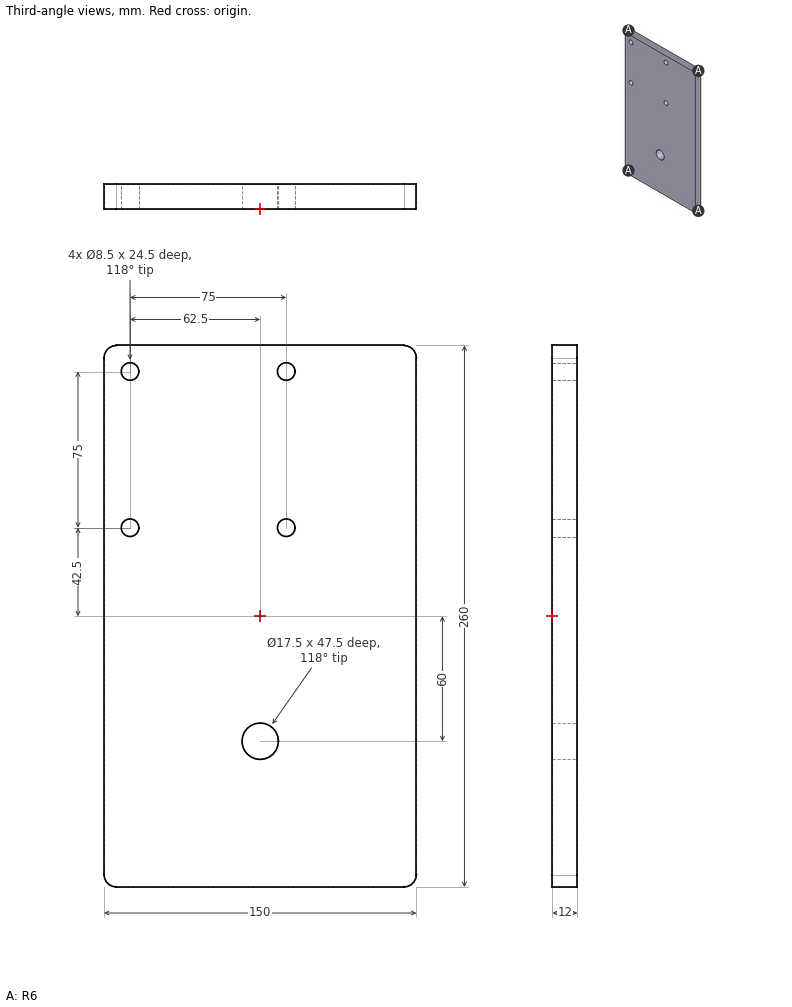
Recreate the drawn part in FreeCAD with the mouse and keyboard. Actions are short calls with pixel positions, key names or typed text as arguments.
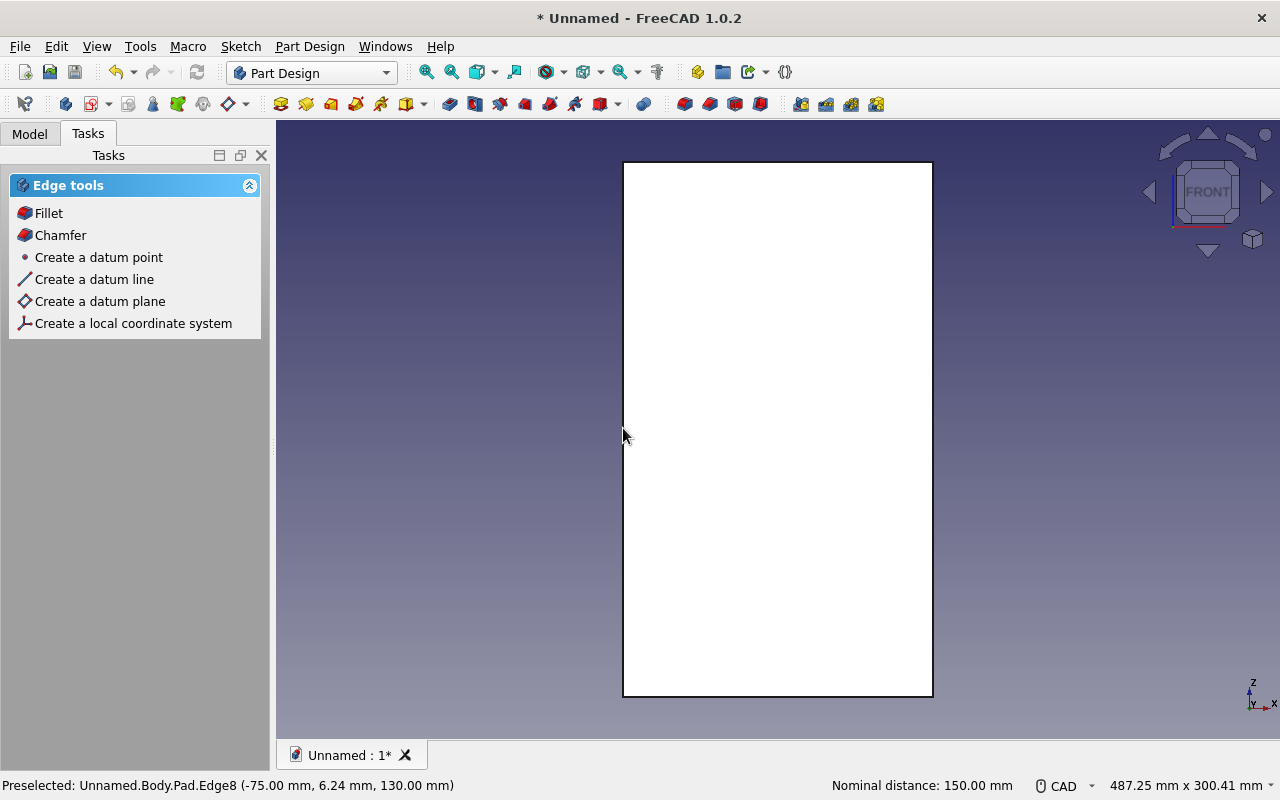
key(3)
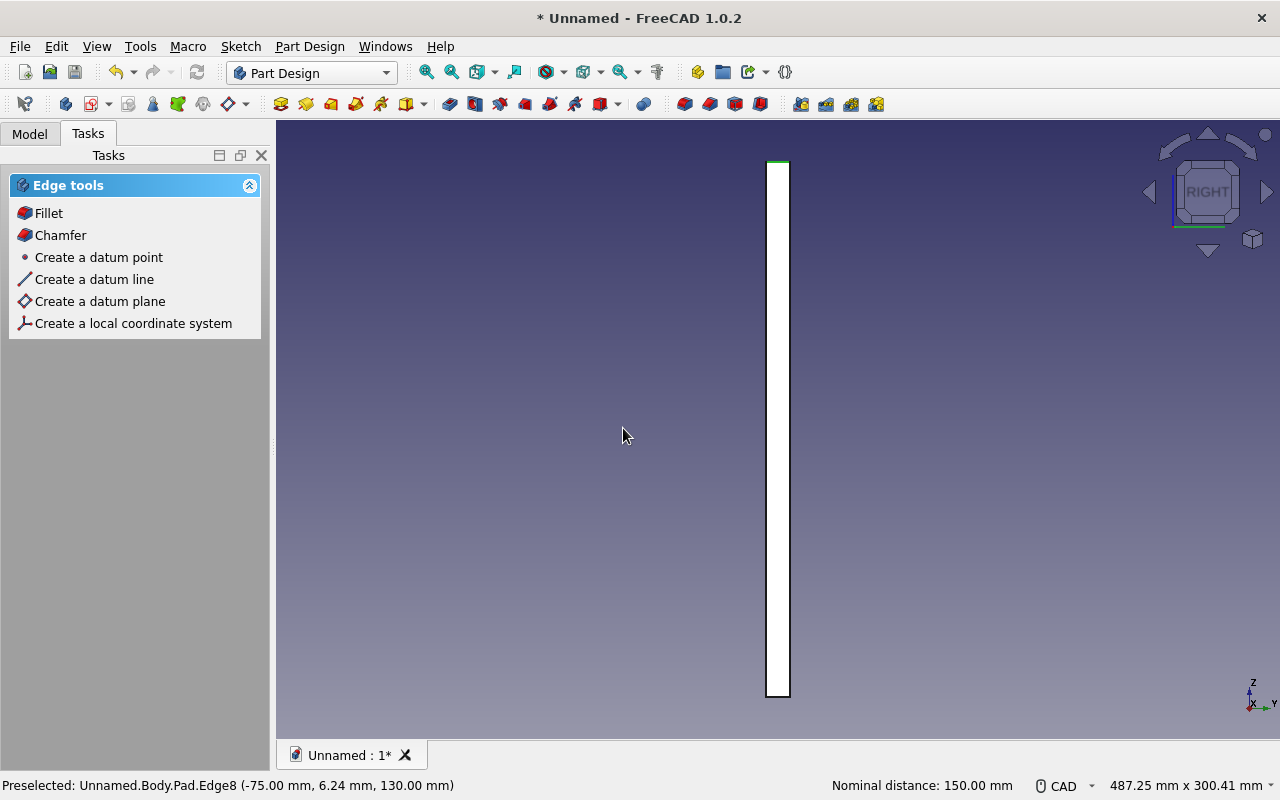
click(778, 696, ctrl)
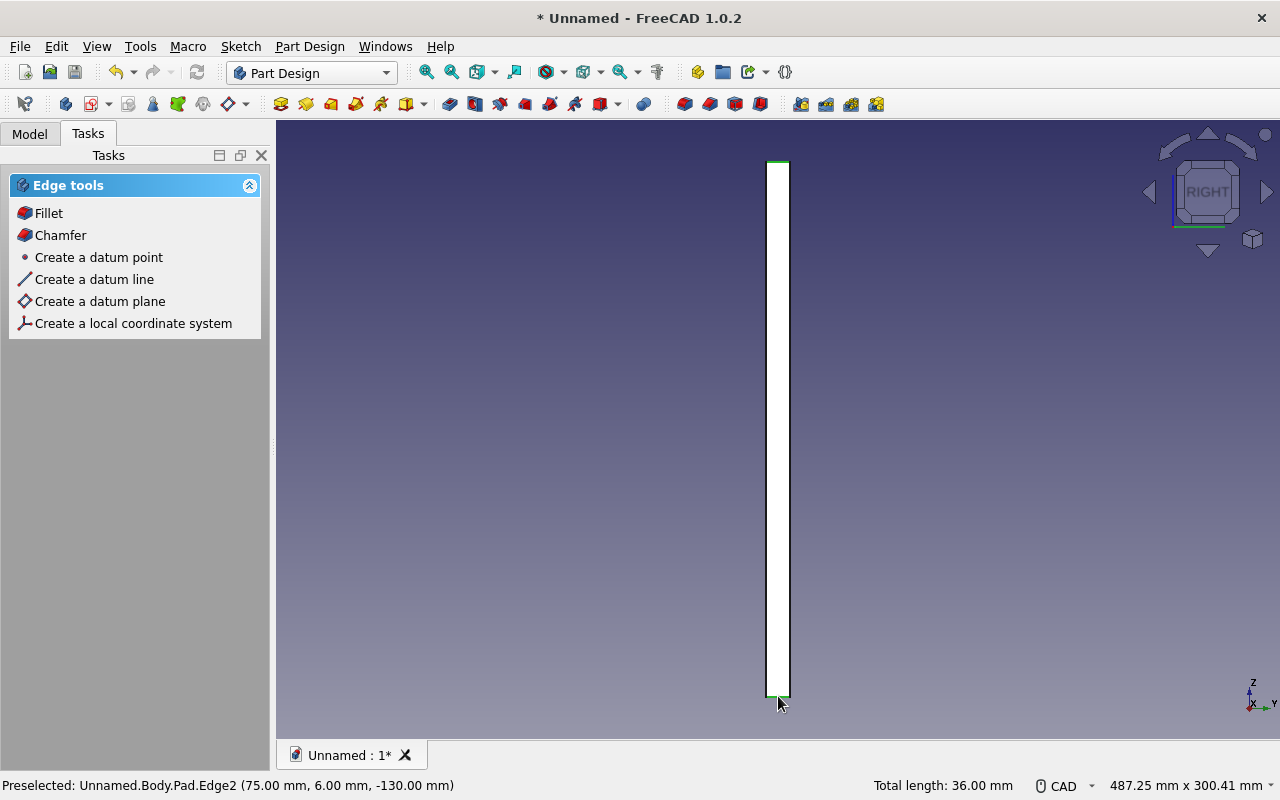
key(5)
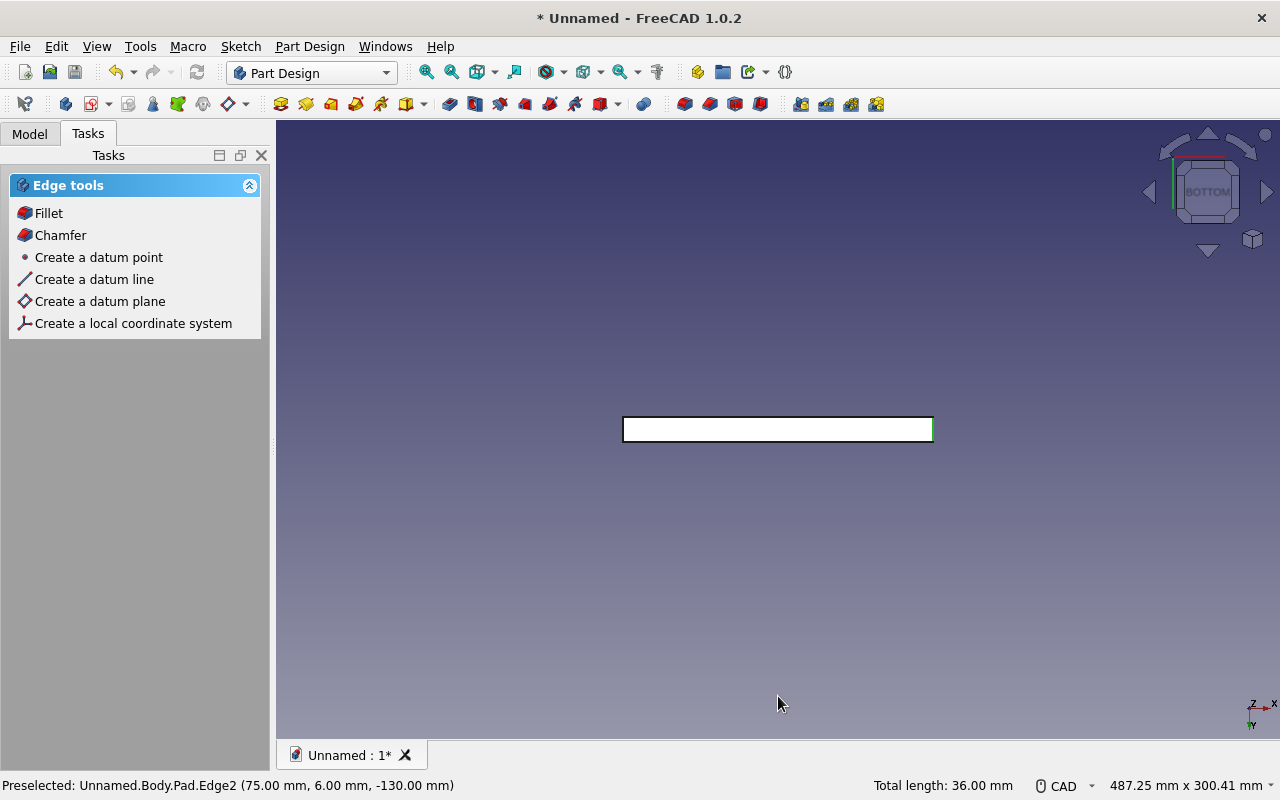
key(v)
key(f)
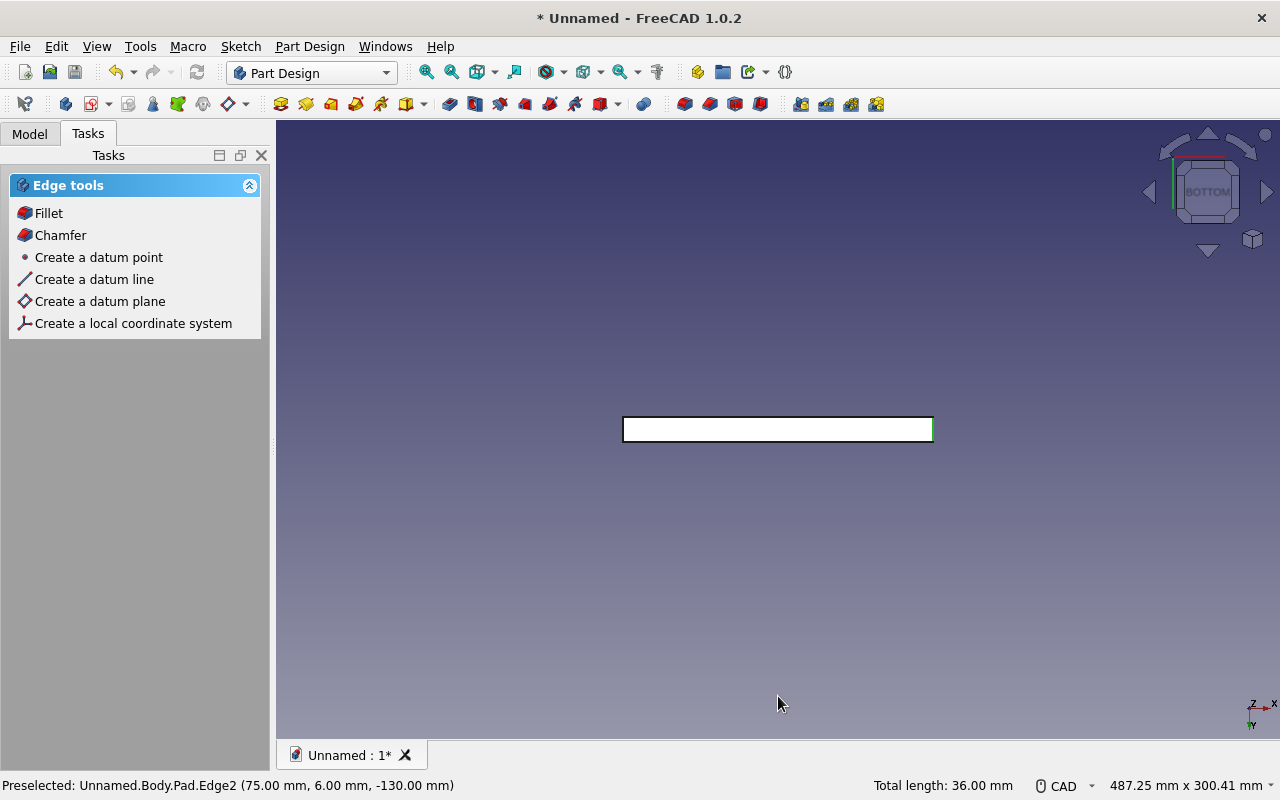
click(623, 428, ctrl)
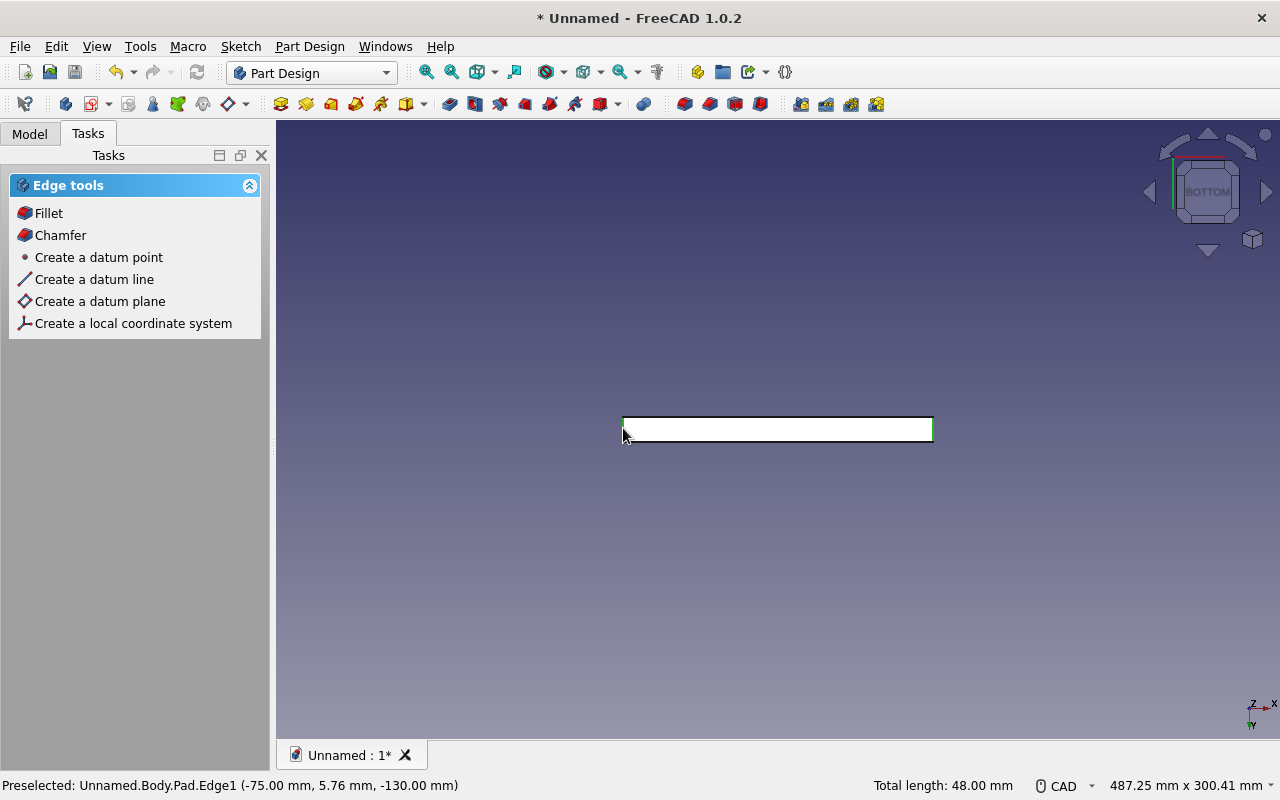
click(685, 104)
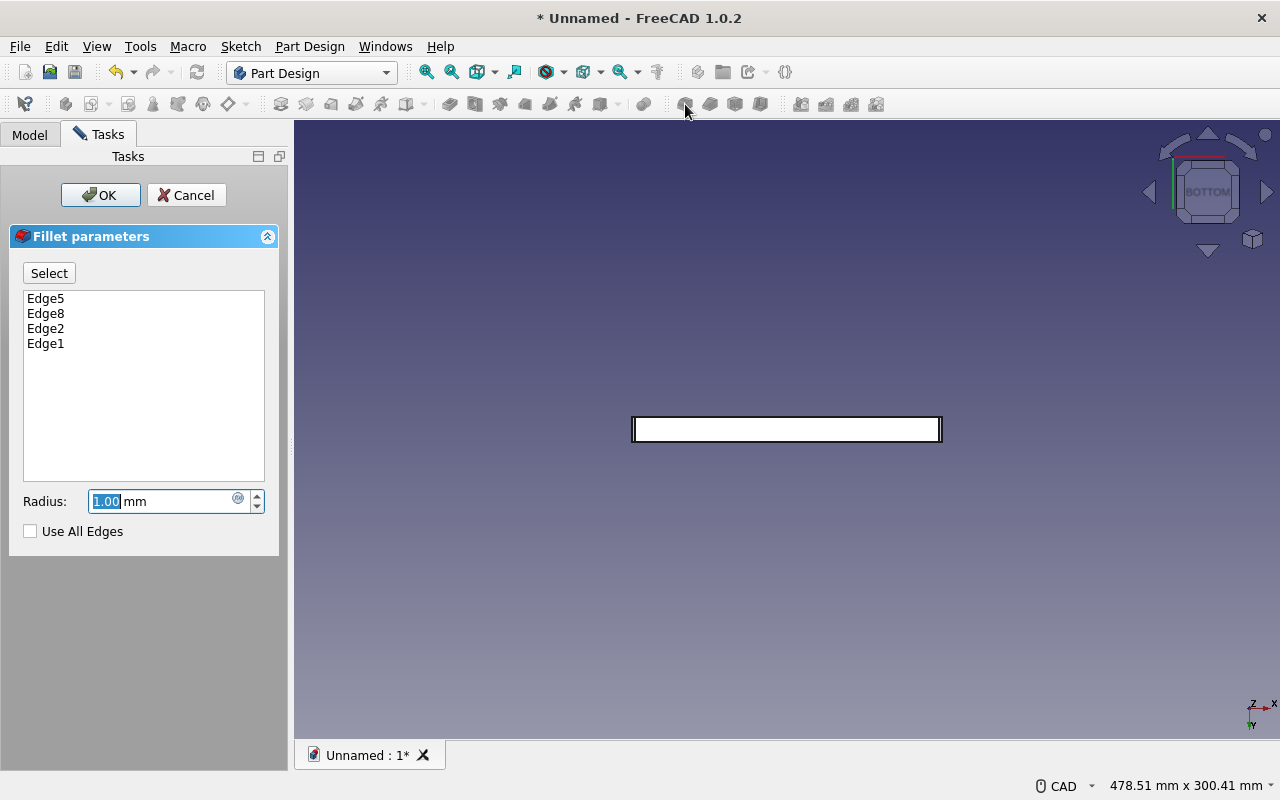
text(6)
key(Tab)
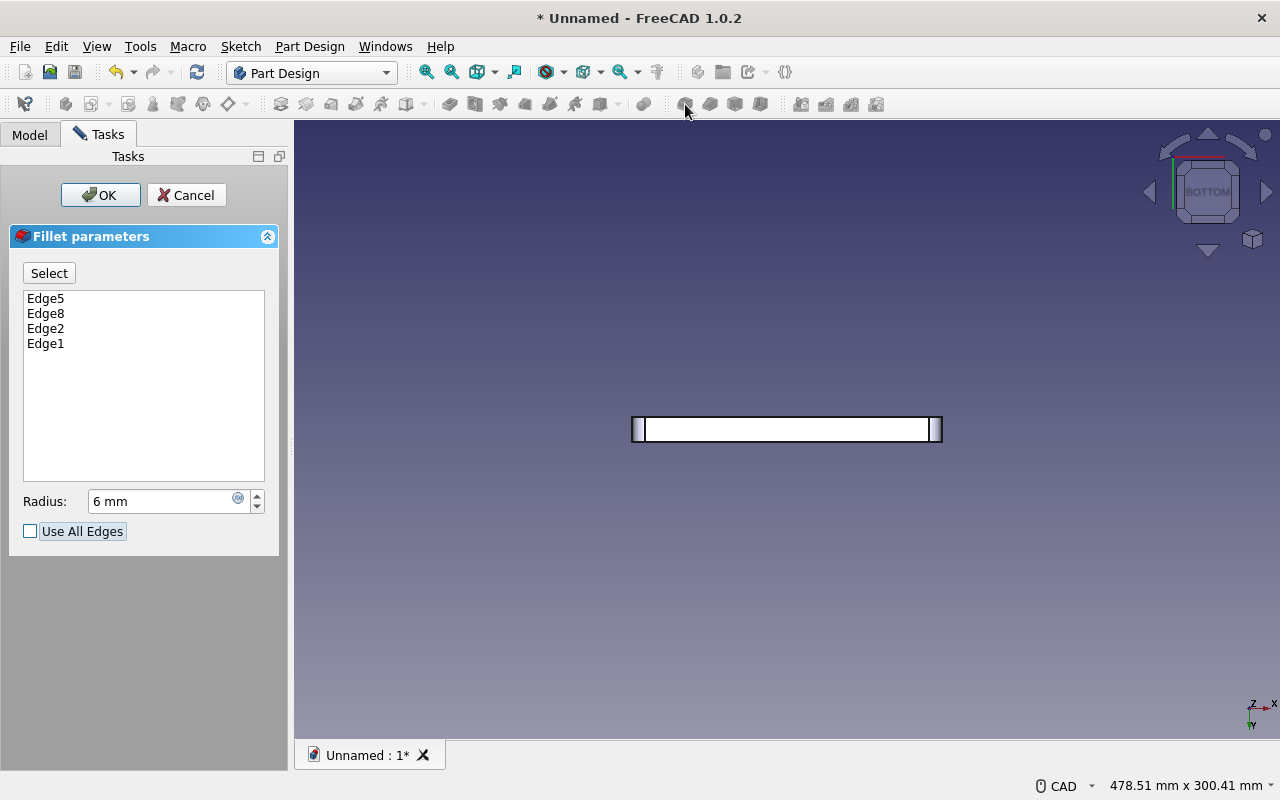
click(101, 195)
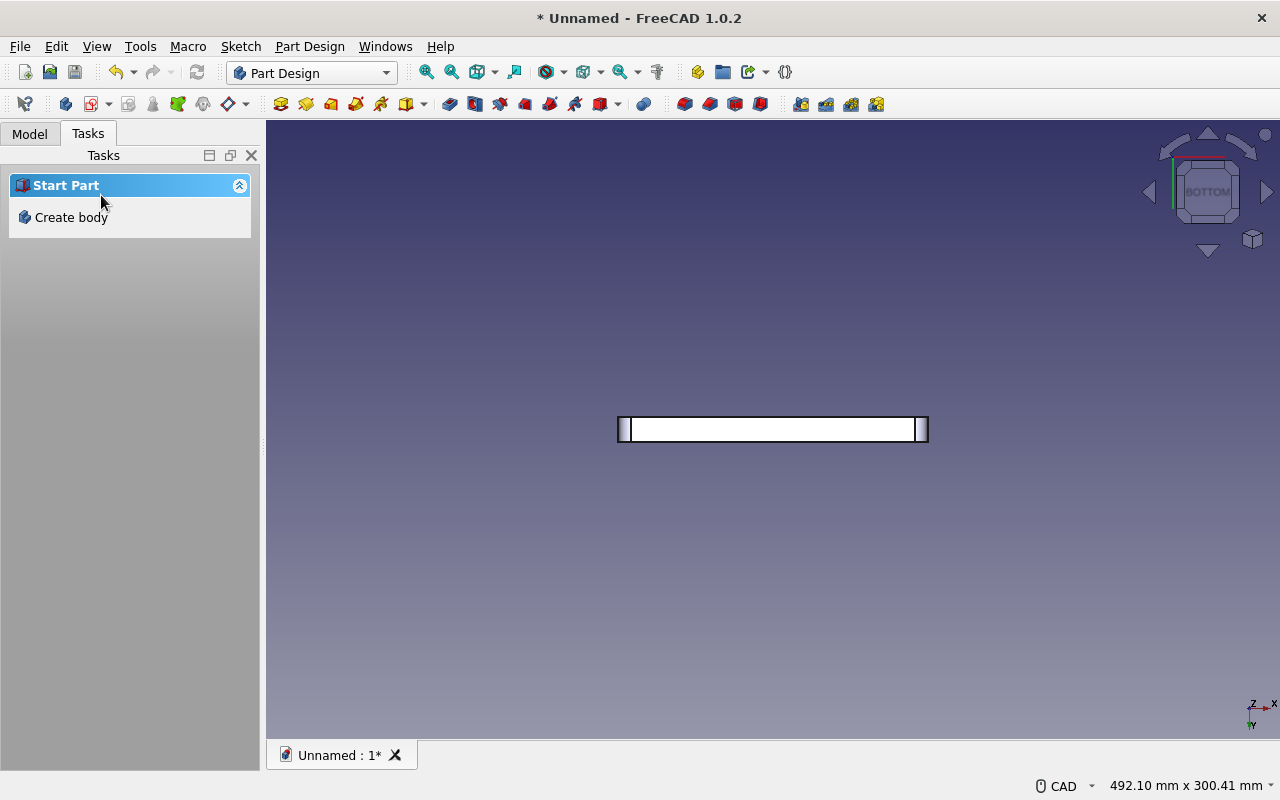
key(v)
key(f)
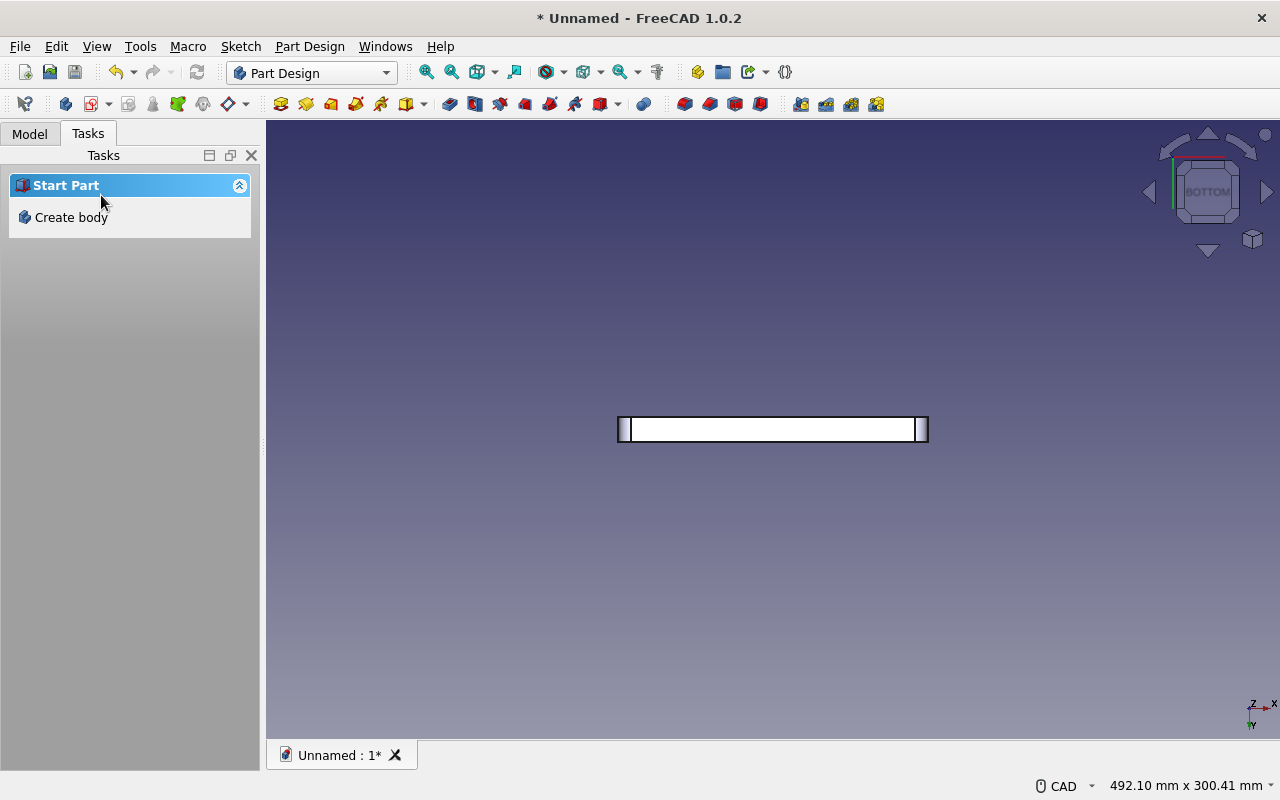
key(0)